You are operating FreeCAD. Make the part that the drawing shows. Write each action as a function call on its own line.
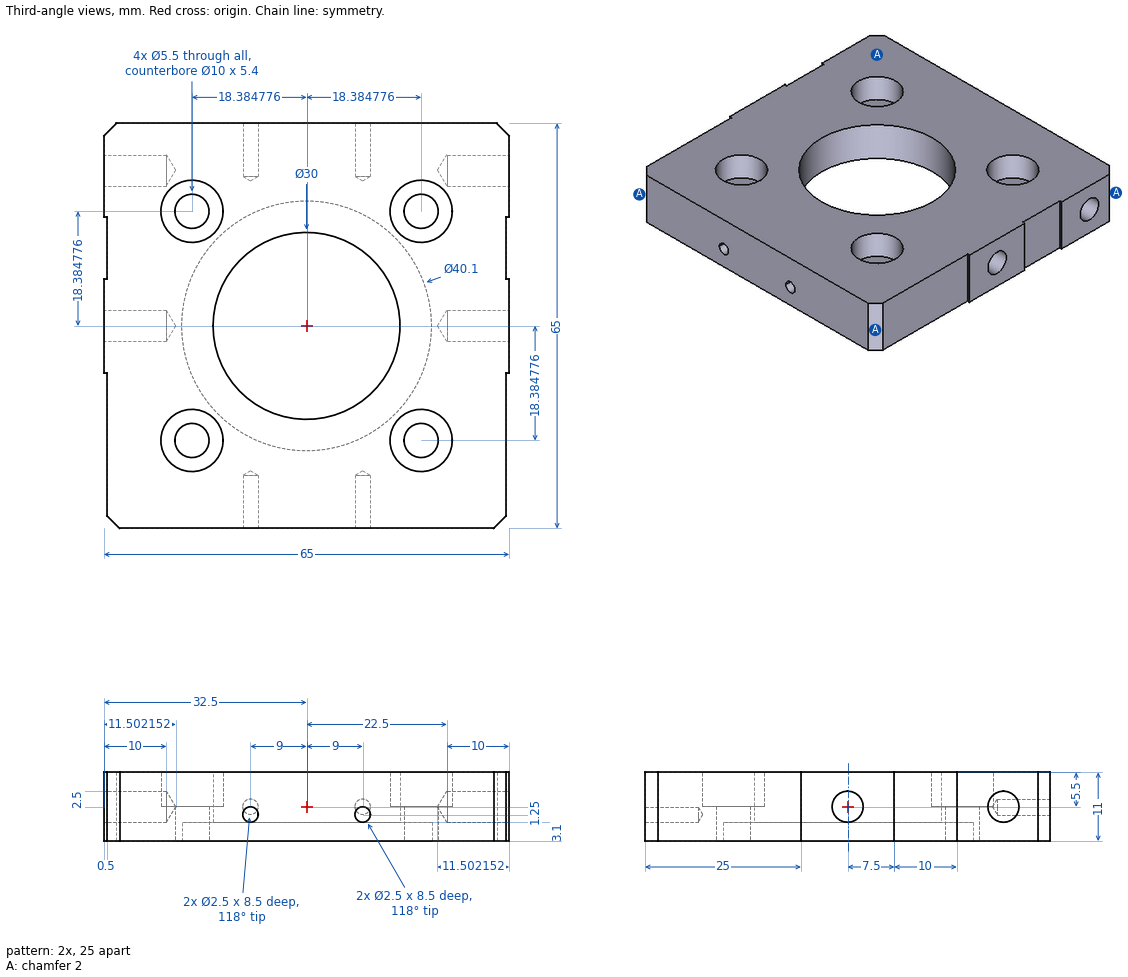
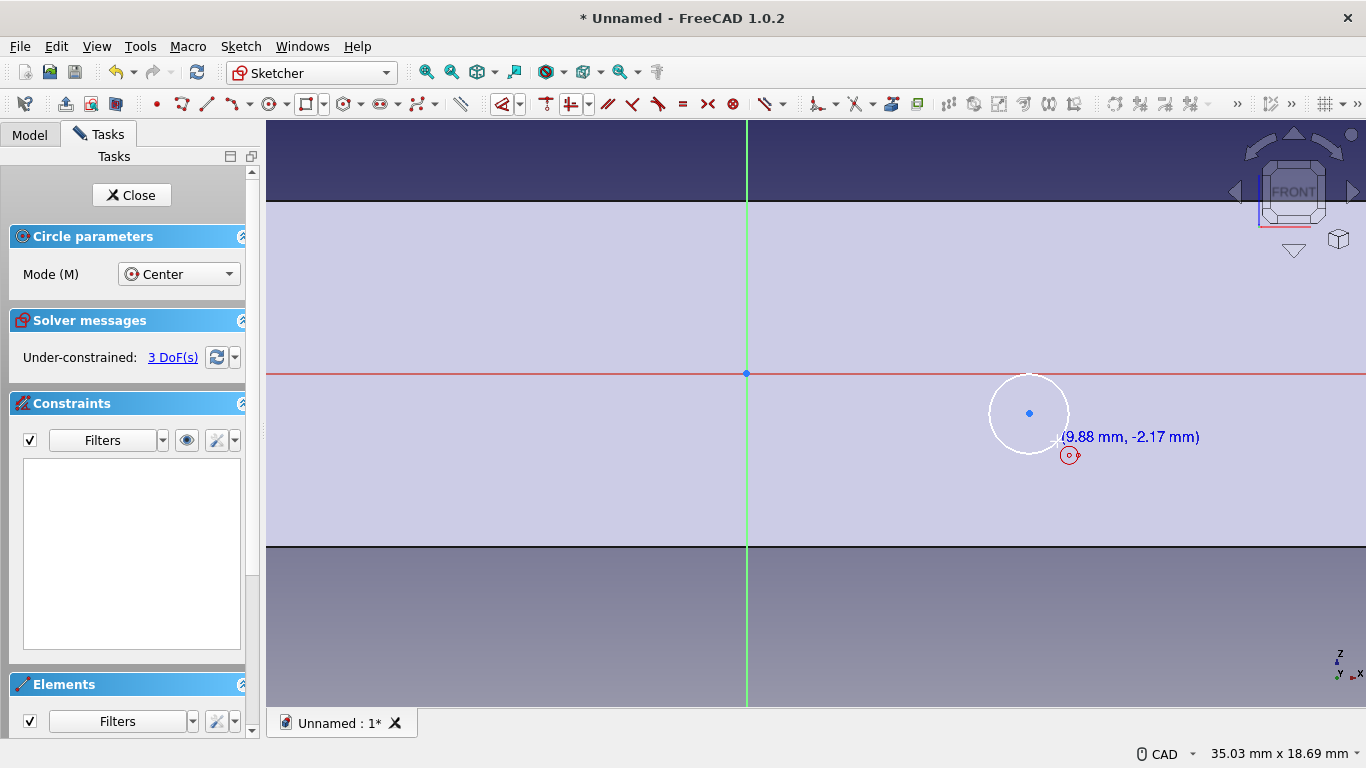
click(464, 413)
click(492, 441)
key(Escape)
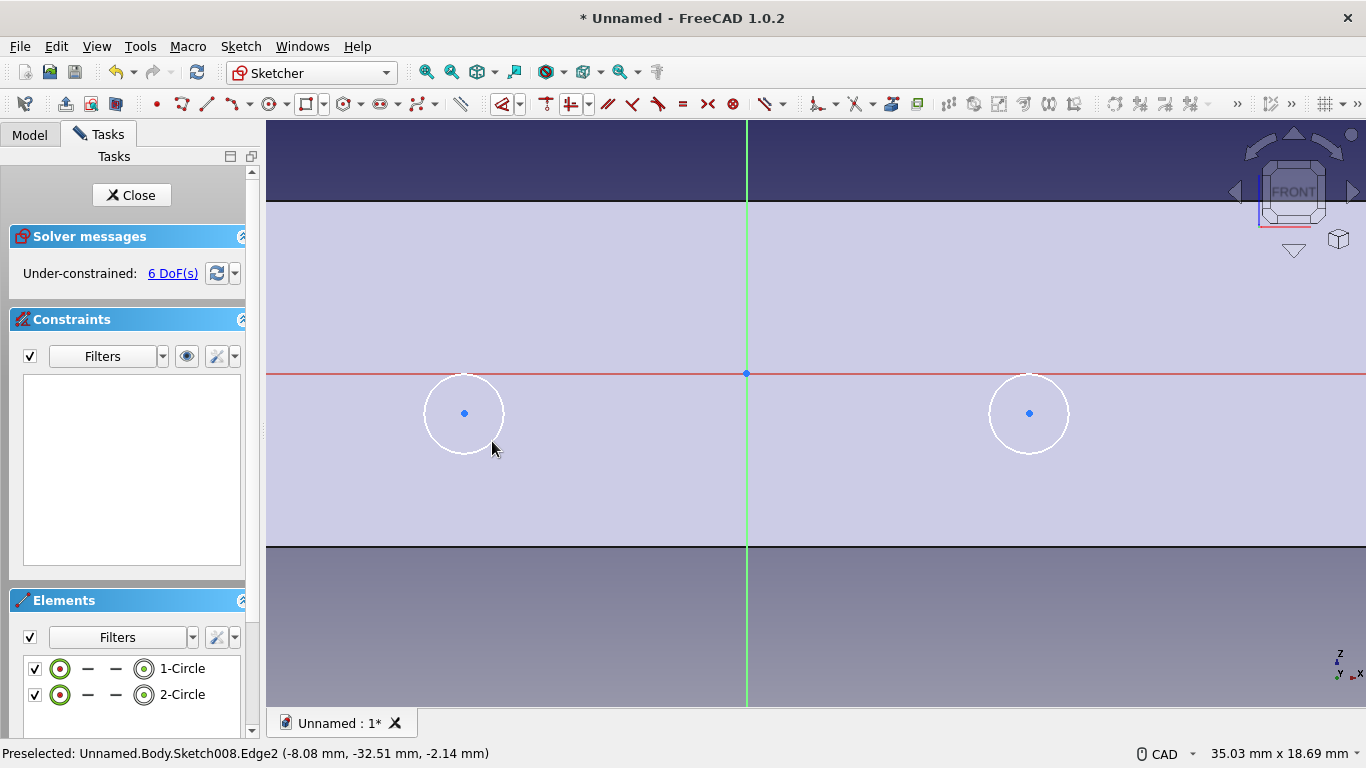
click(1057, 386)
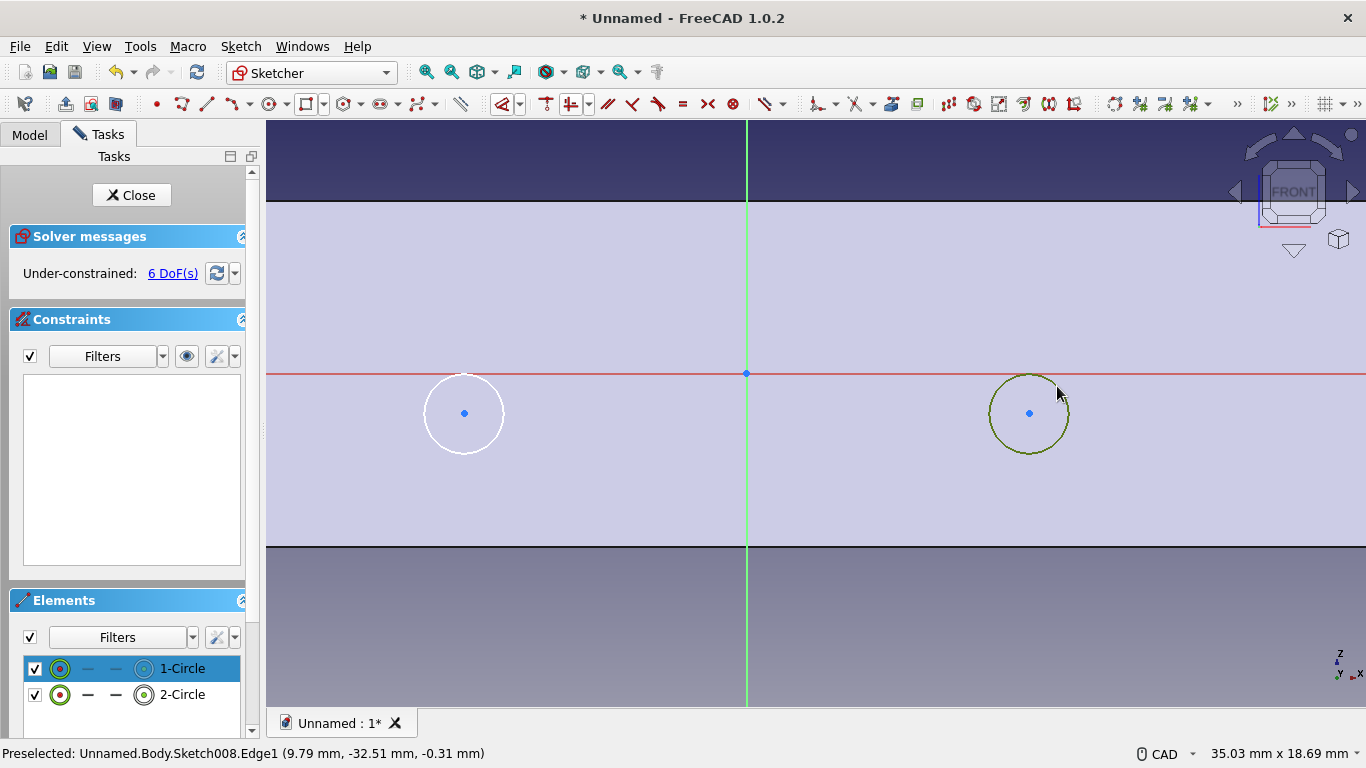
click(492, 386)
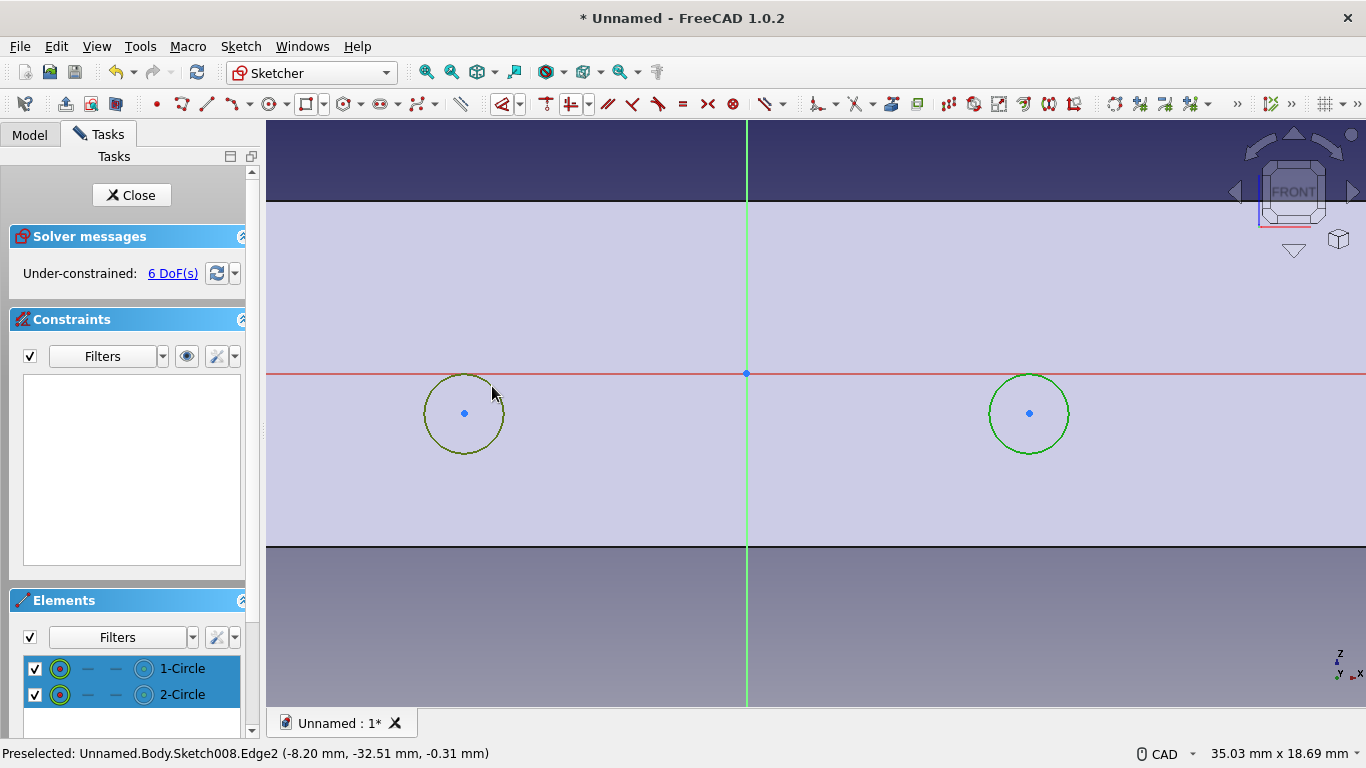
click(683, 104)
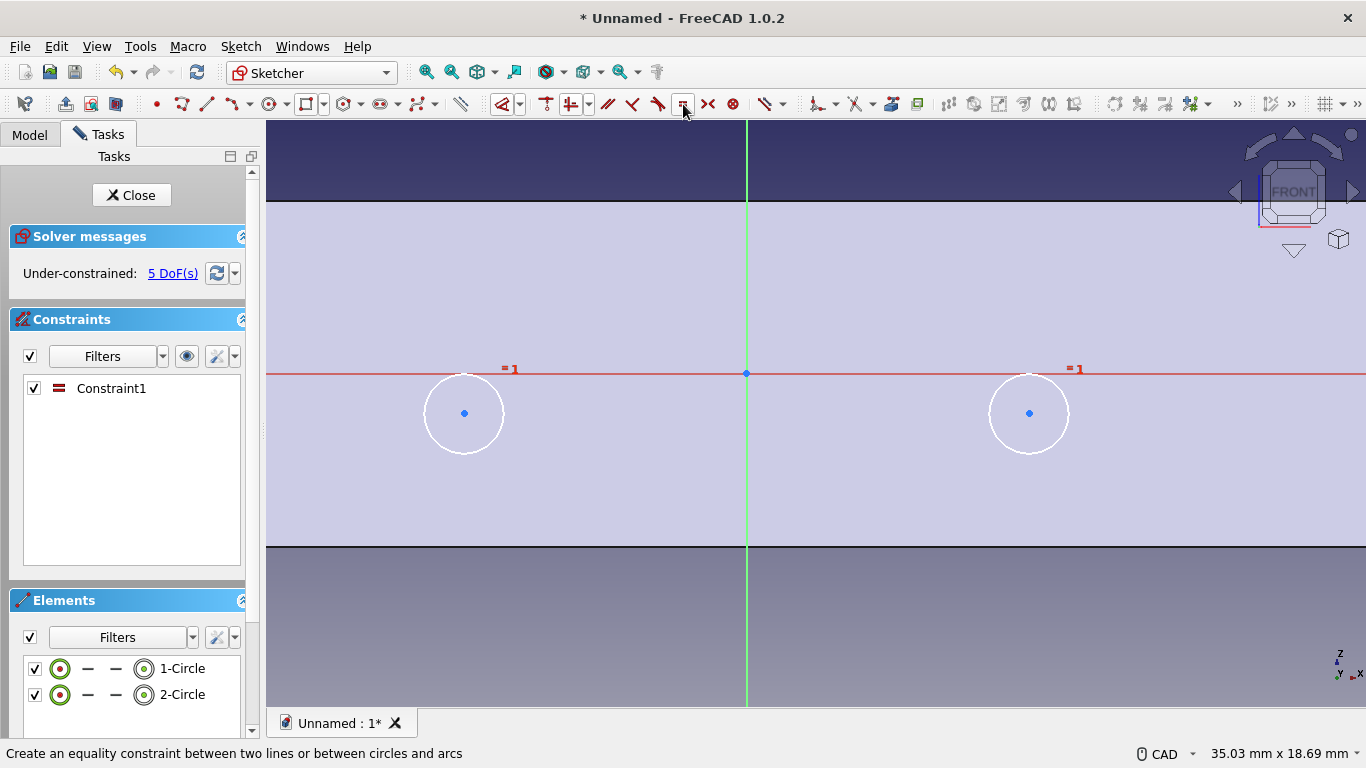
click(1029, 414)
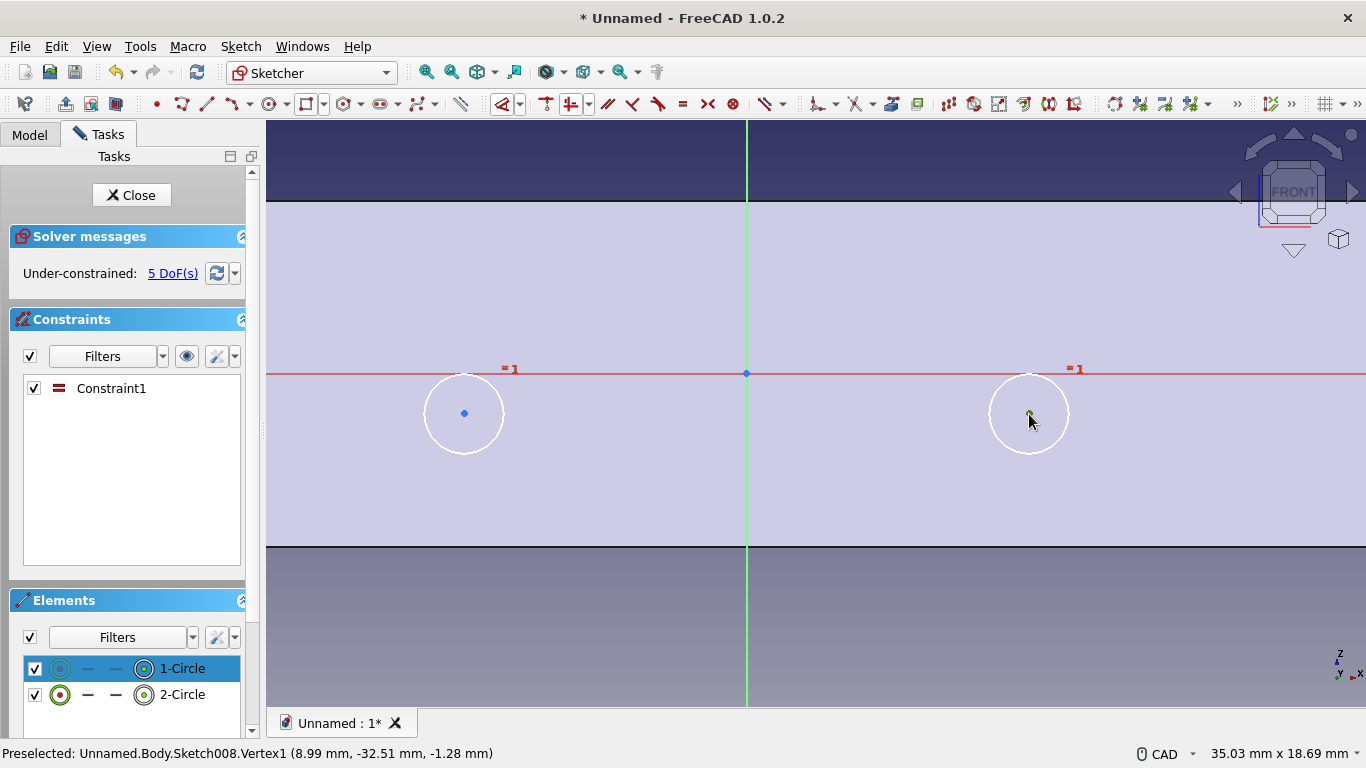
click(464, 414)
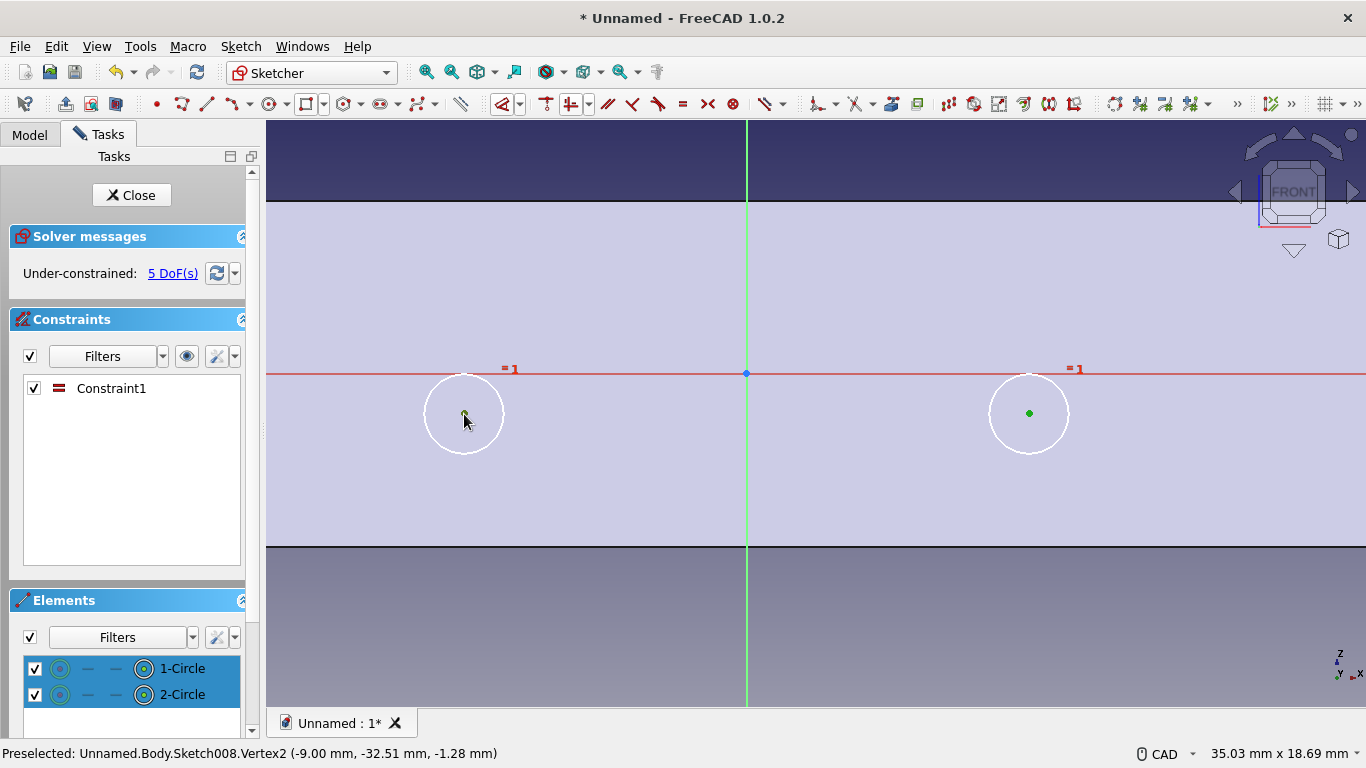
click(588, 104)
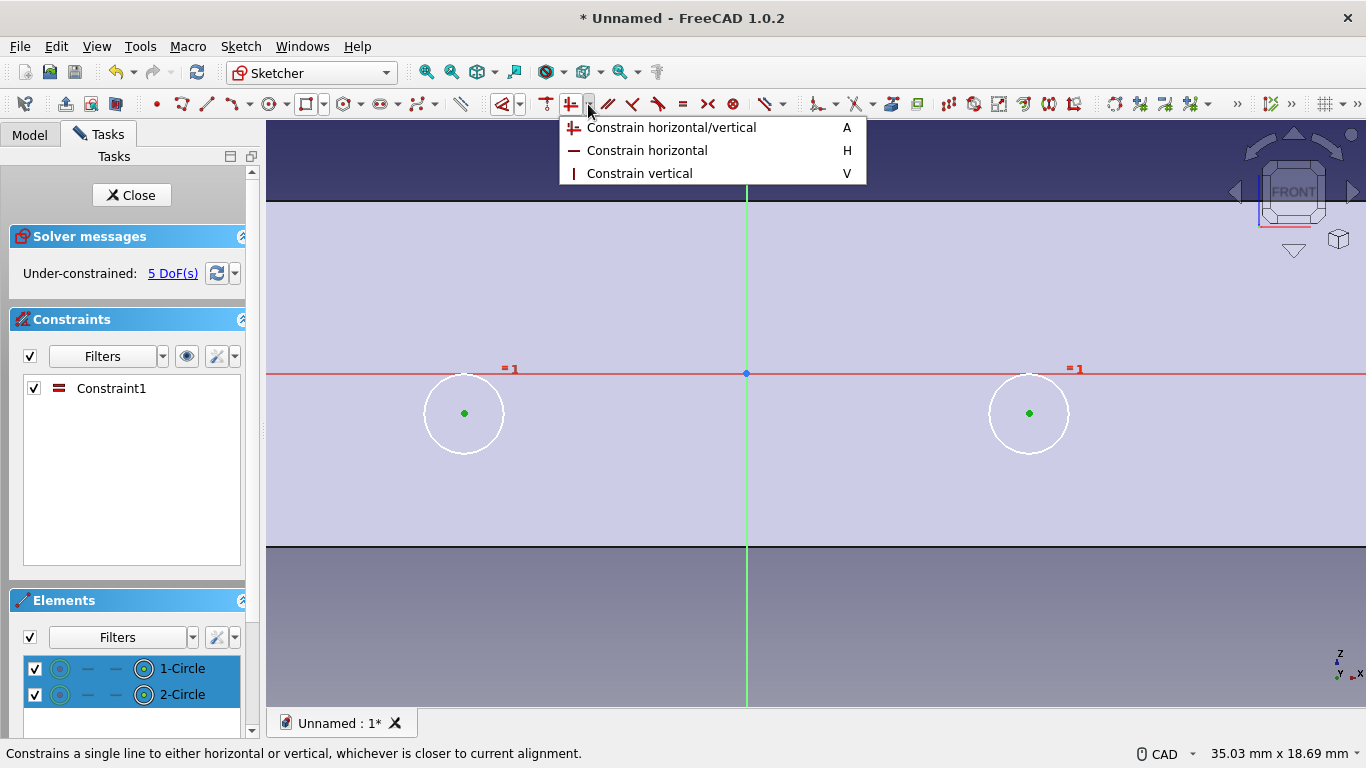
click(713, 150)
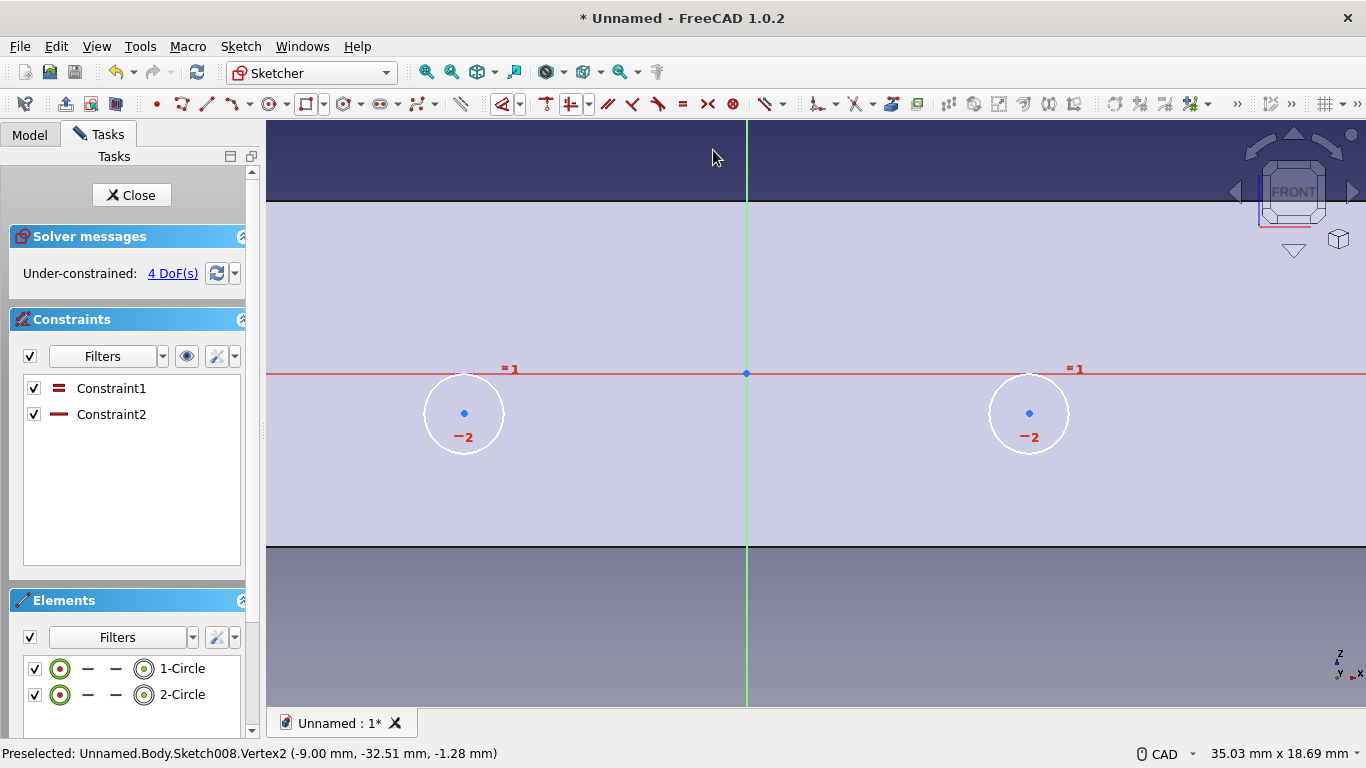
click(1057, 386)